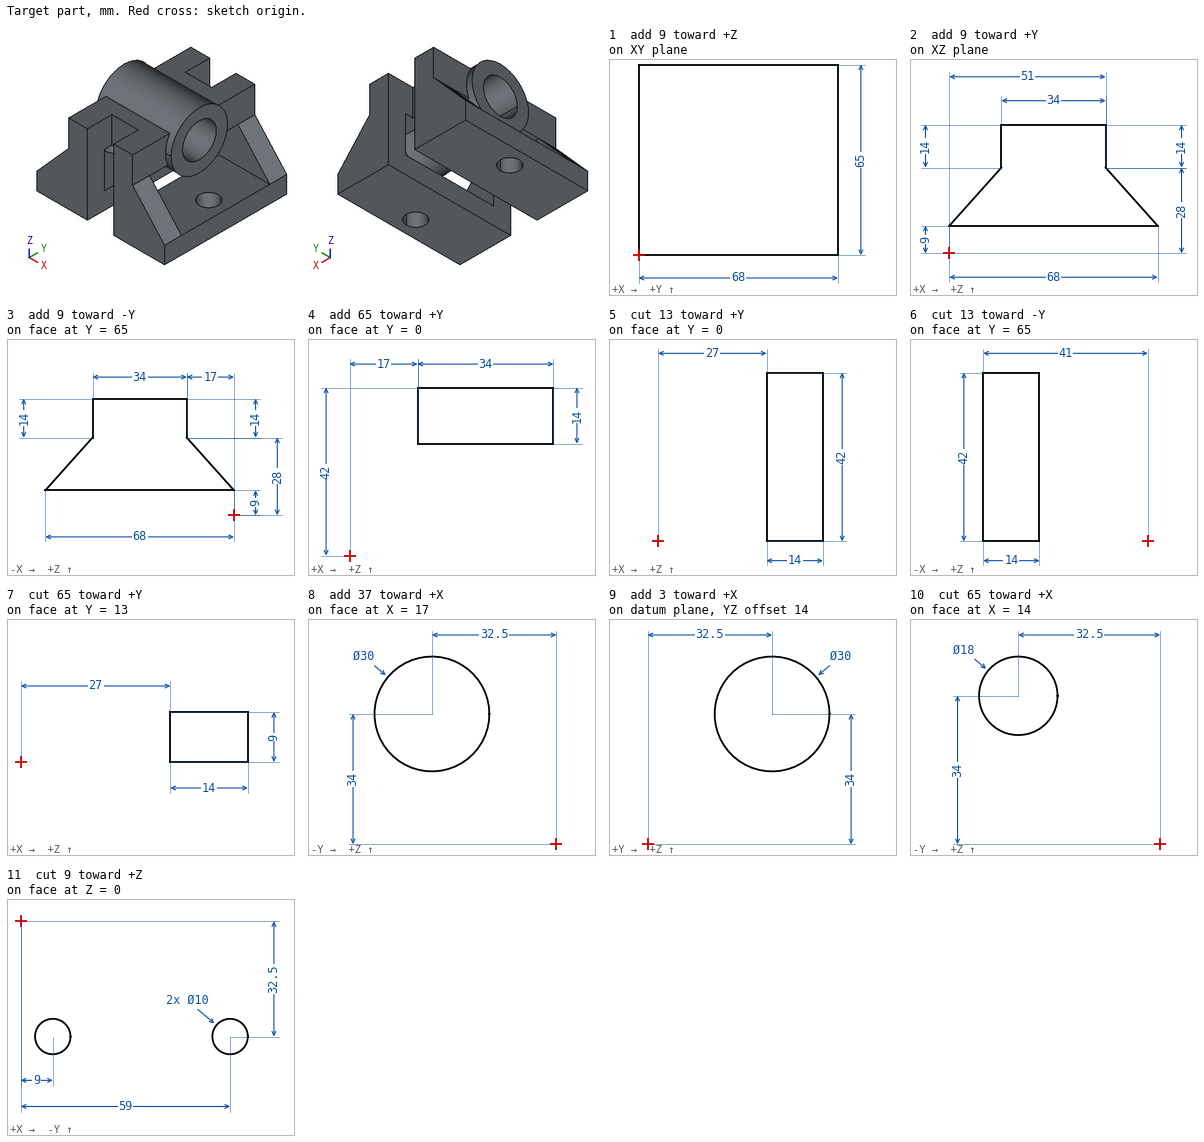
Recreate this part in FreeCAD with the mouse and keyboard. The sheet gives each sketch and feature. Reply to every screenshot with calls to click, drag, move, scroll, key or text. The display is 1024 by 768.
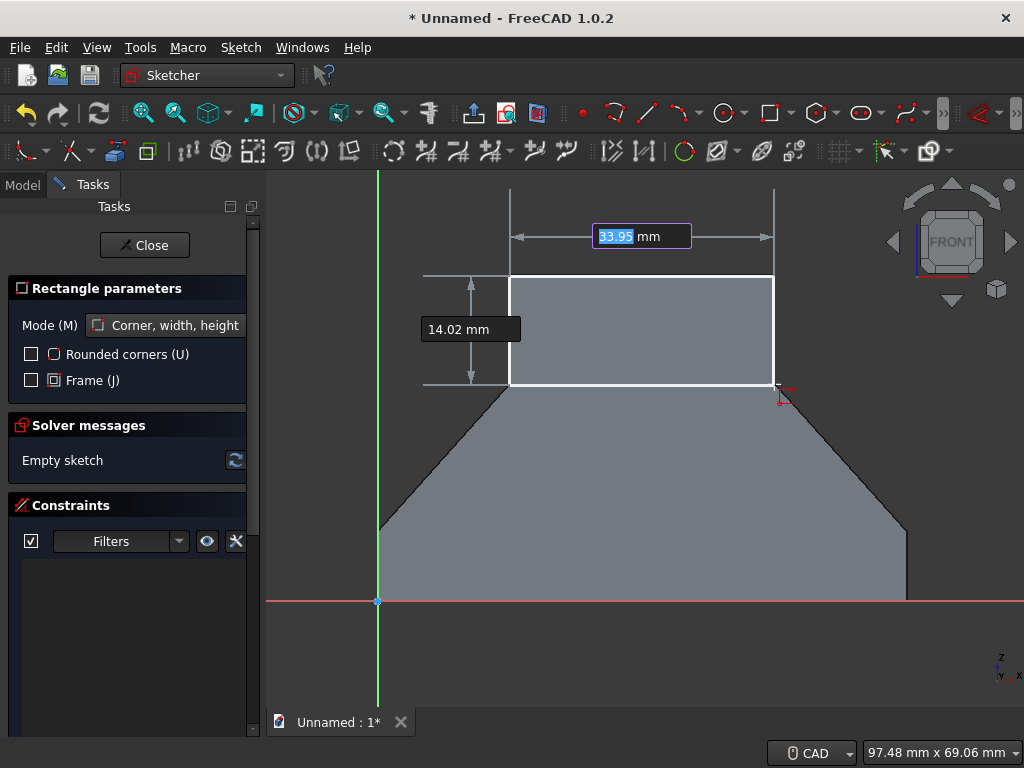
text(34)
key(Tab)
text(14)
key(Return)
key(Escape)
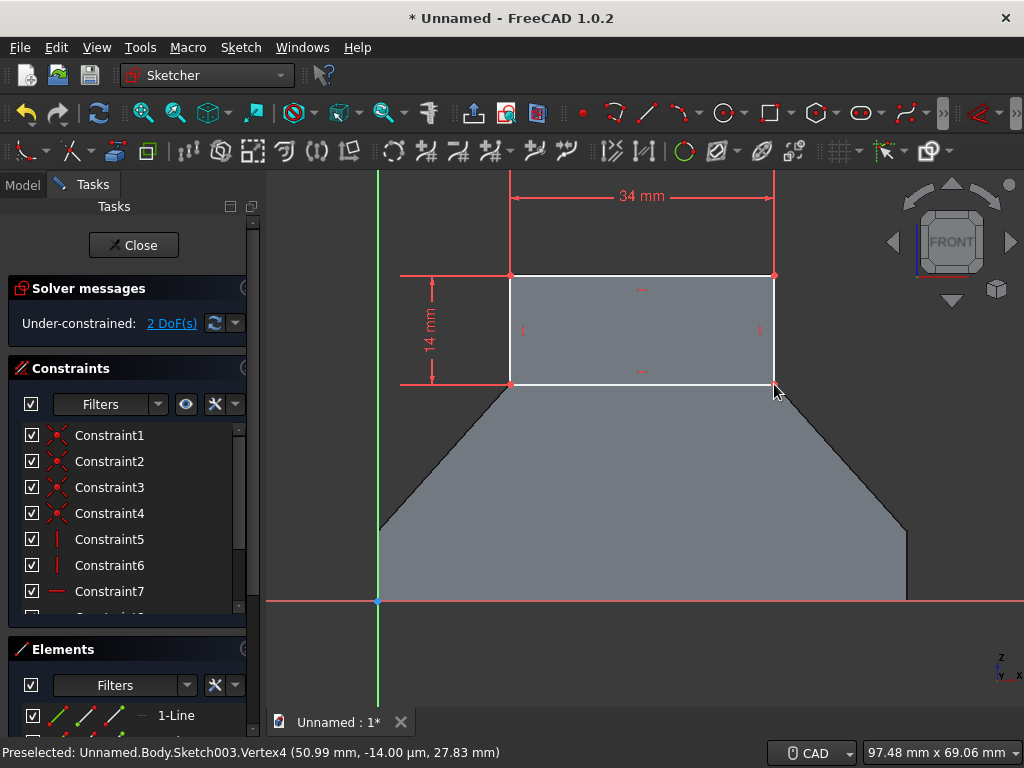
click(978, 114)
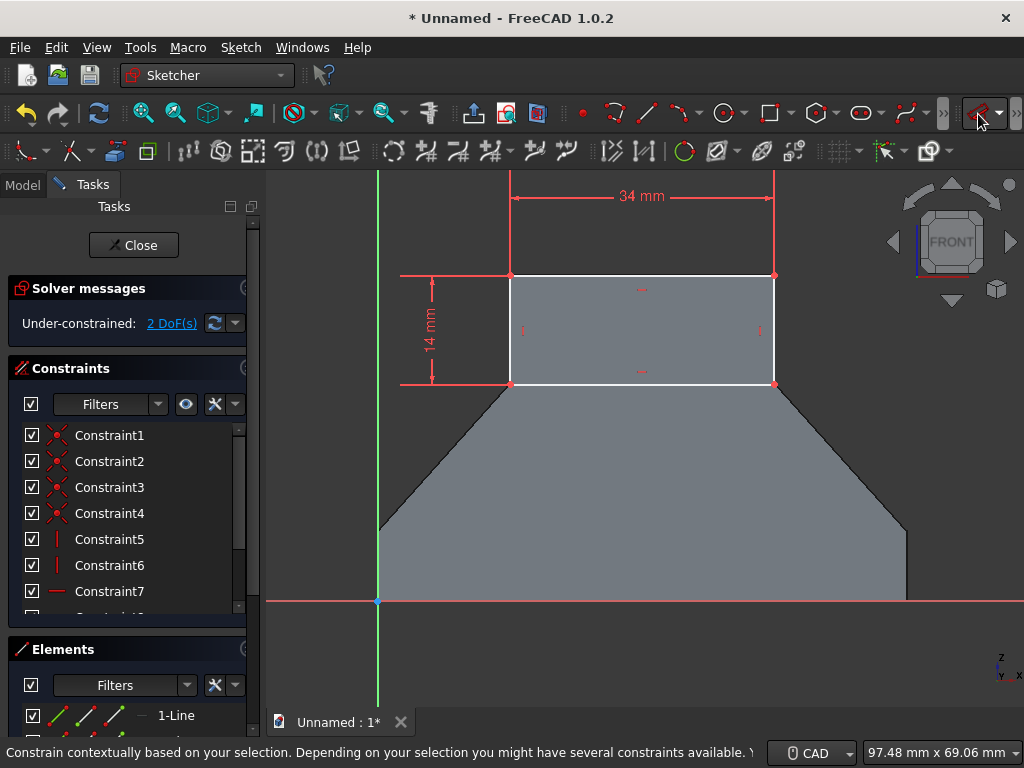
click(510, 276)
click(444, 635)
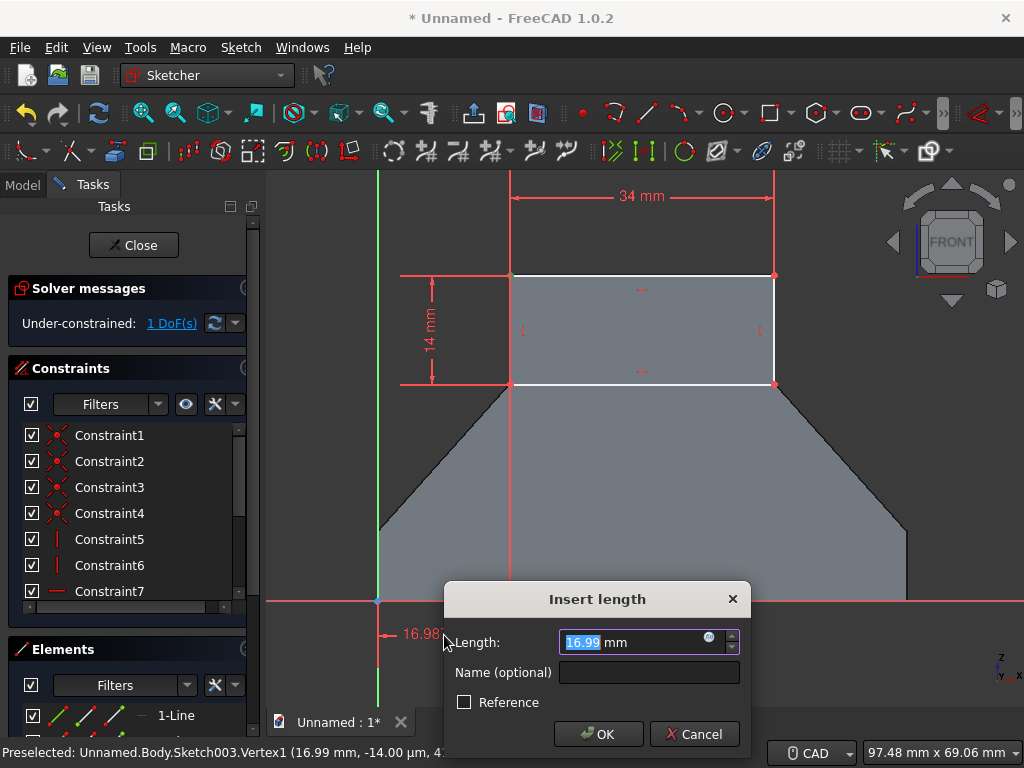
text(17)
key(Return)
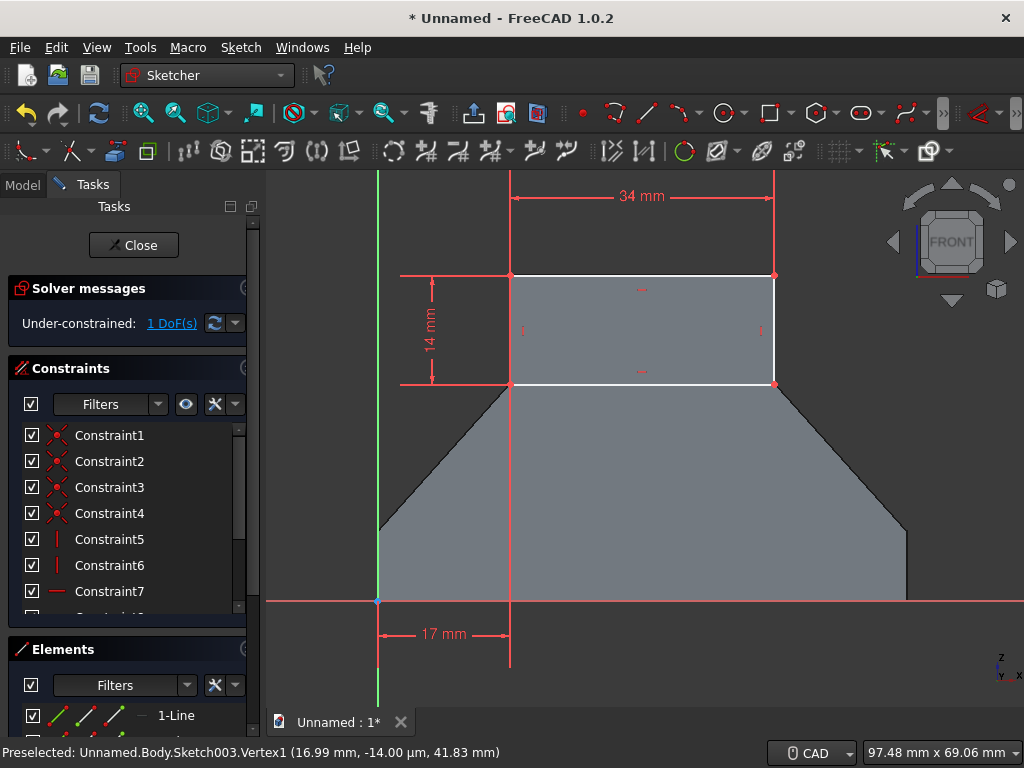
click(510, 276)
click(344, 439)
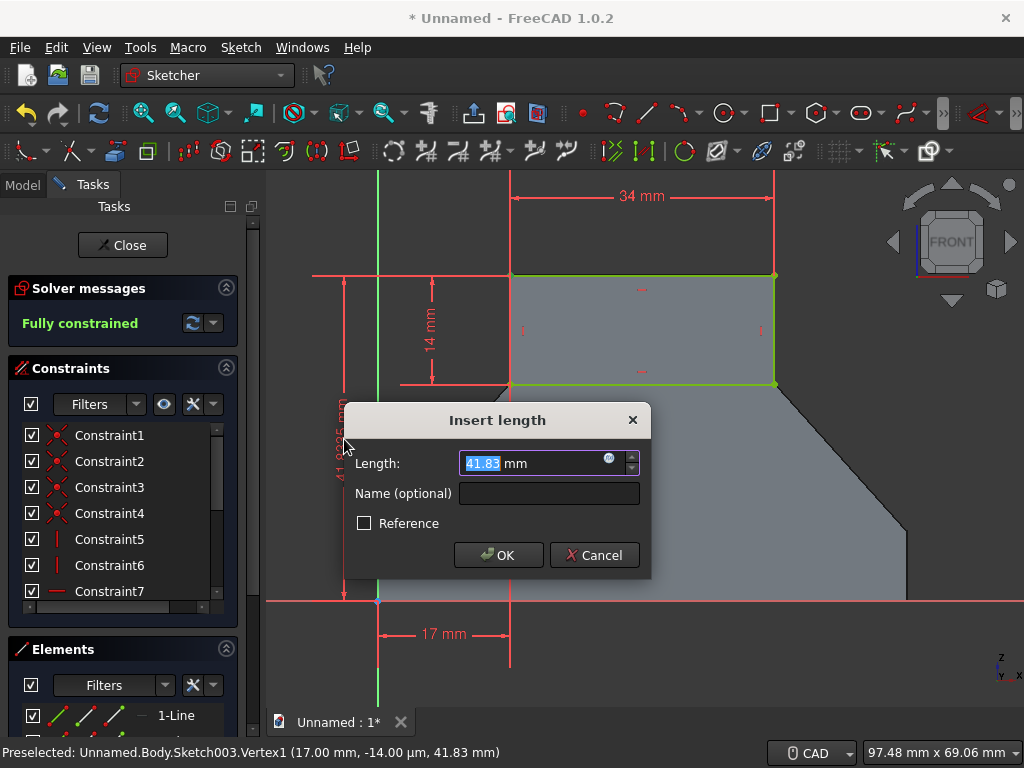
text(42)
key(Return)
key(Escape)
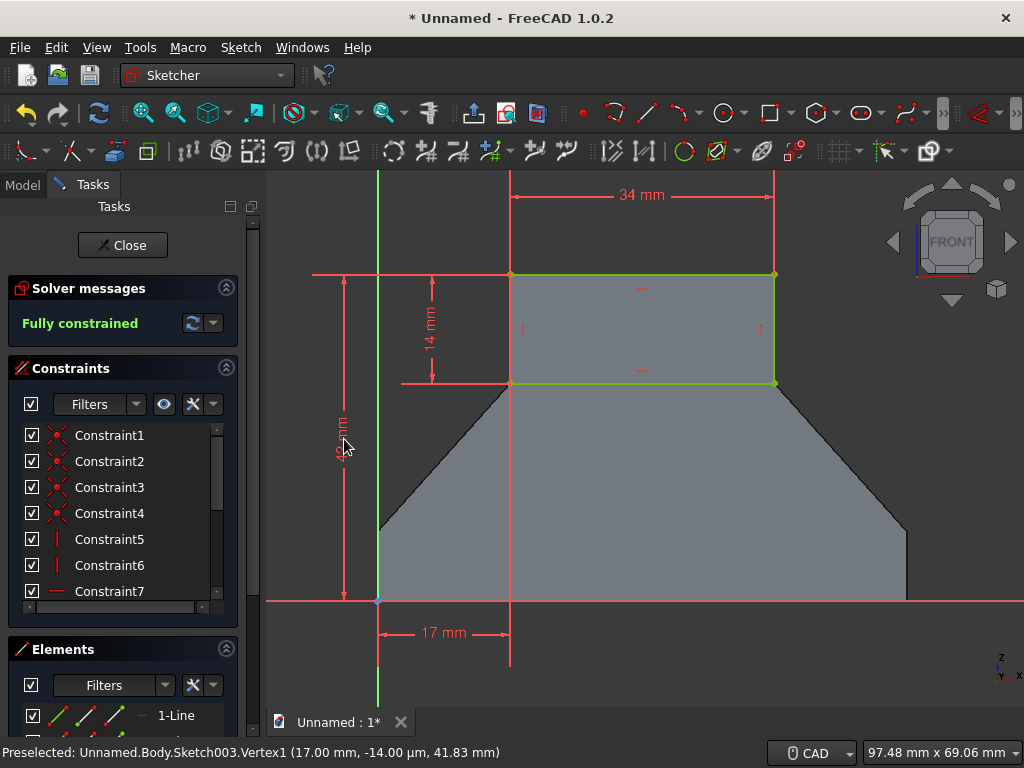
click(123, 245)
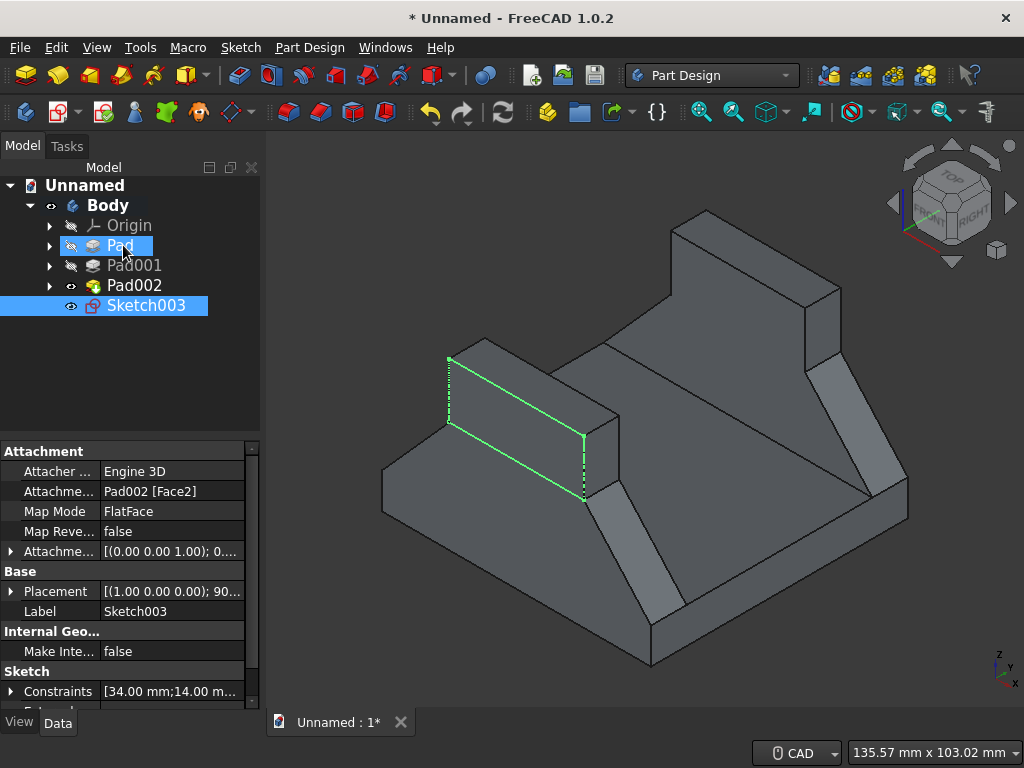
click(26, 76)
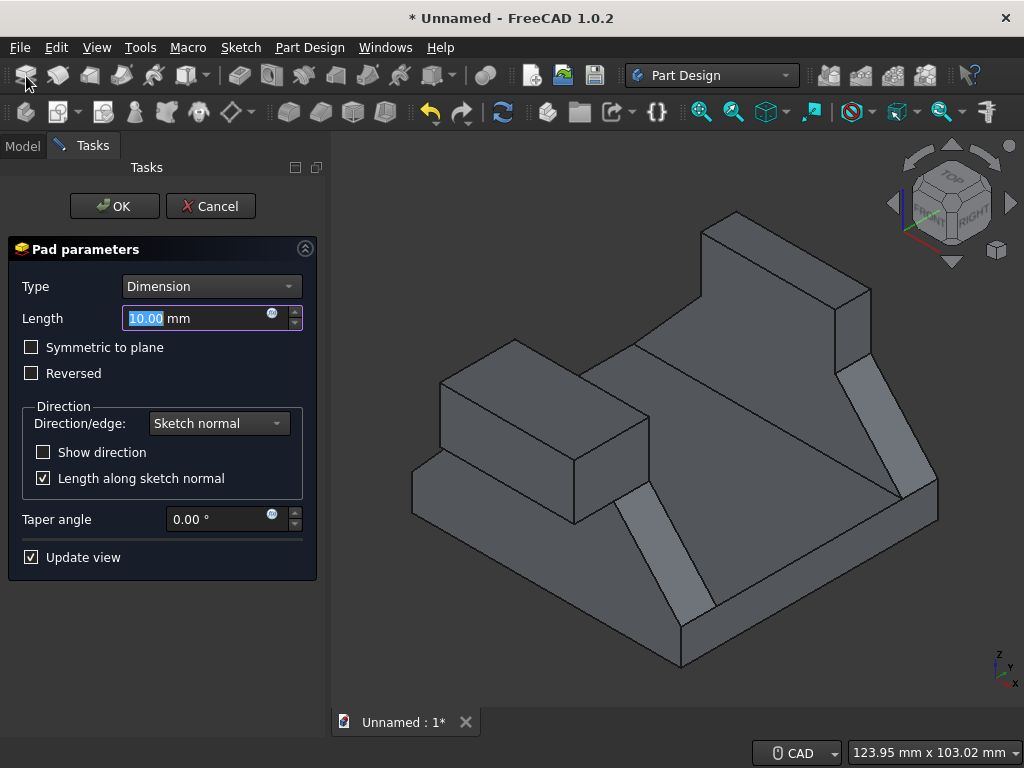
text(65)
key(Tab)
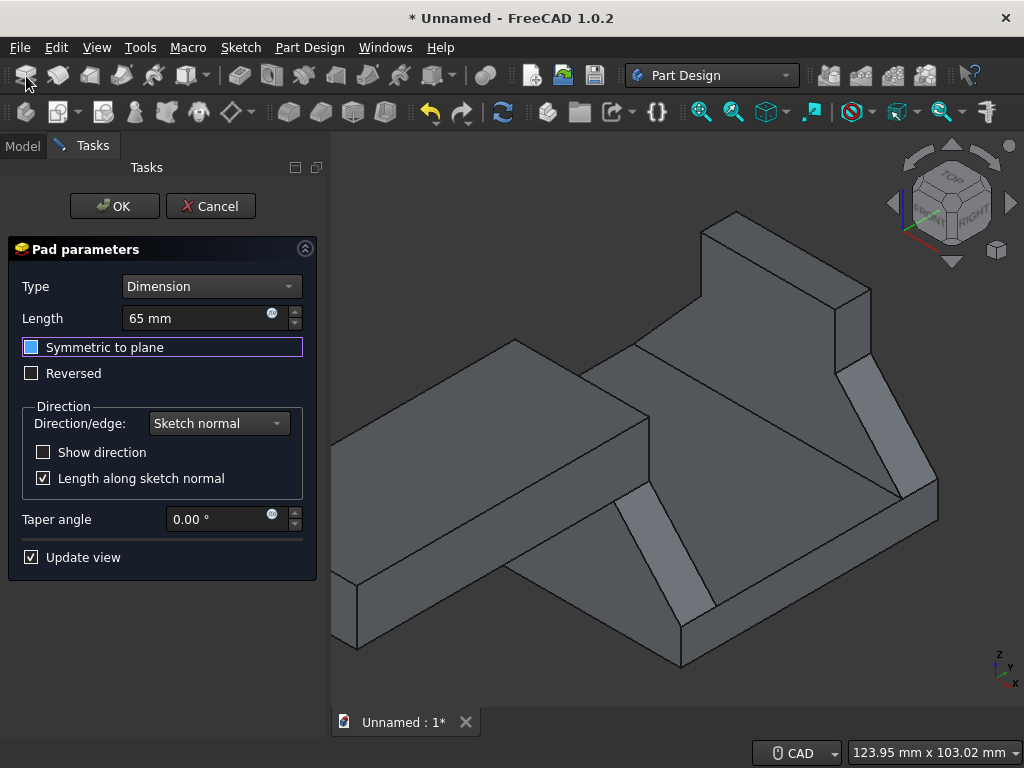
click(30, 373)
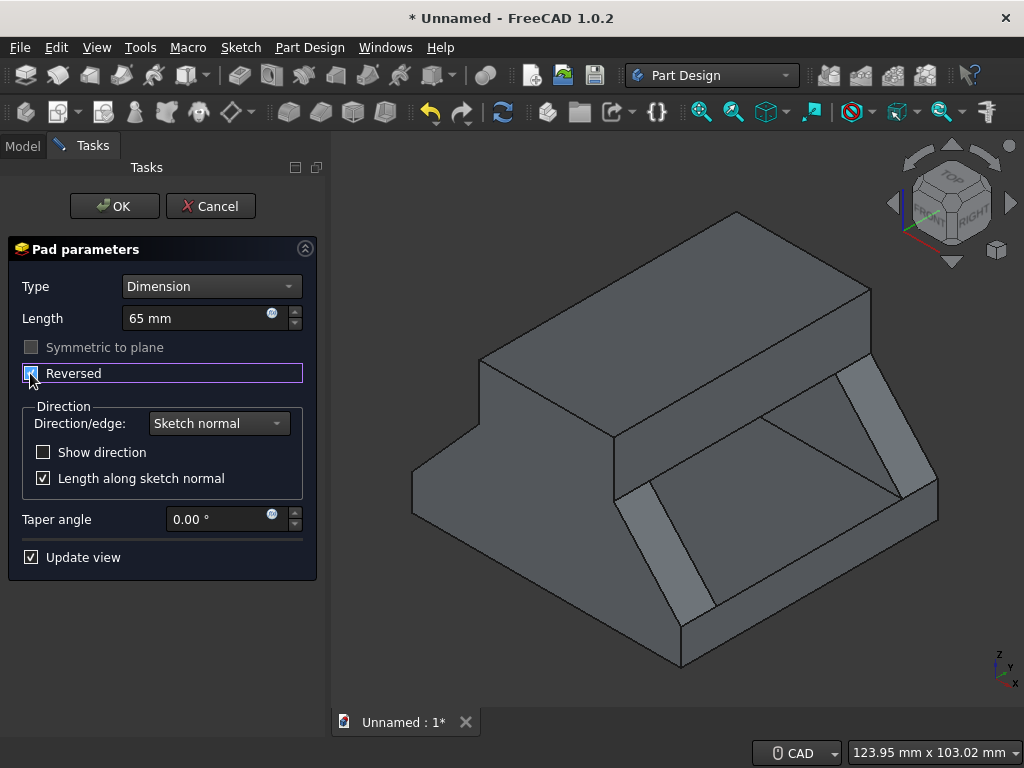
click(115, 206)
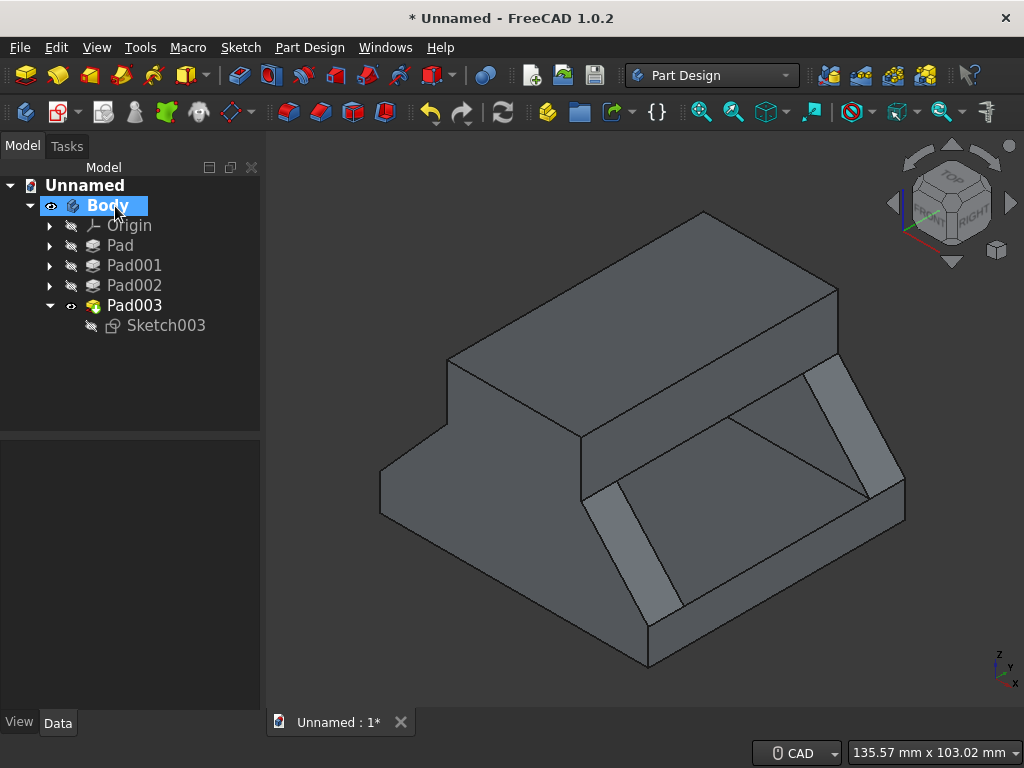
click(514, 494)